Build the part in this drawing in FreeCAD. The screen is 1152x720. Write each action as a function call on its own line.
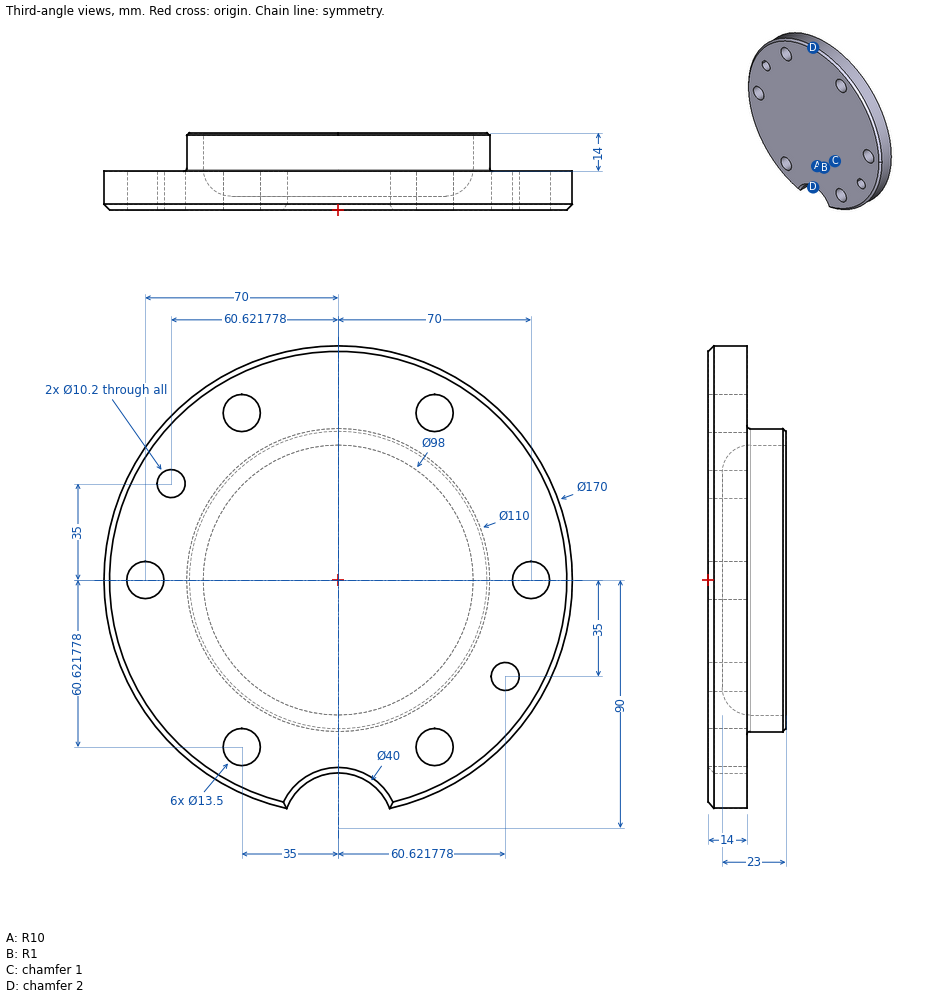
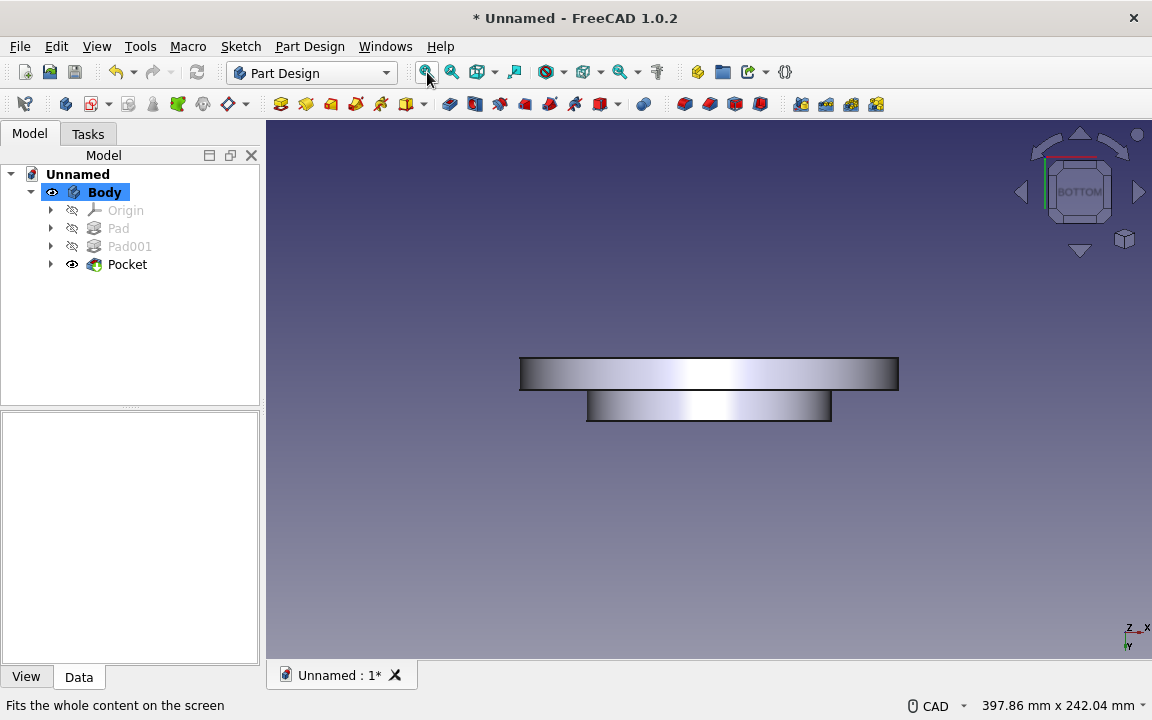
click(427, 72)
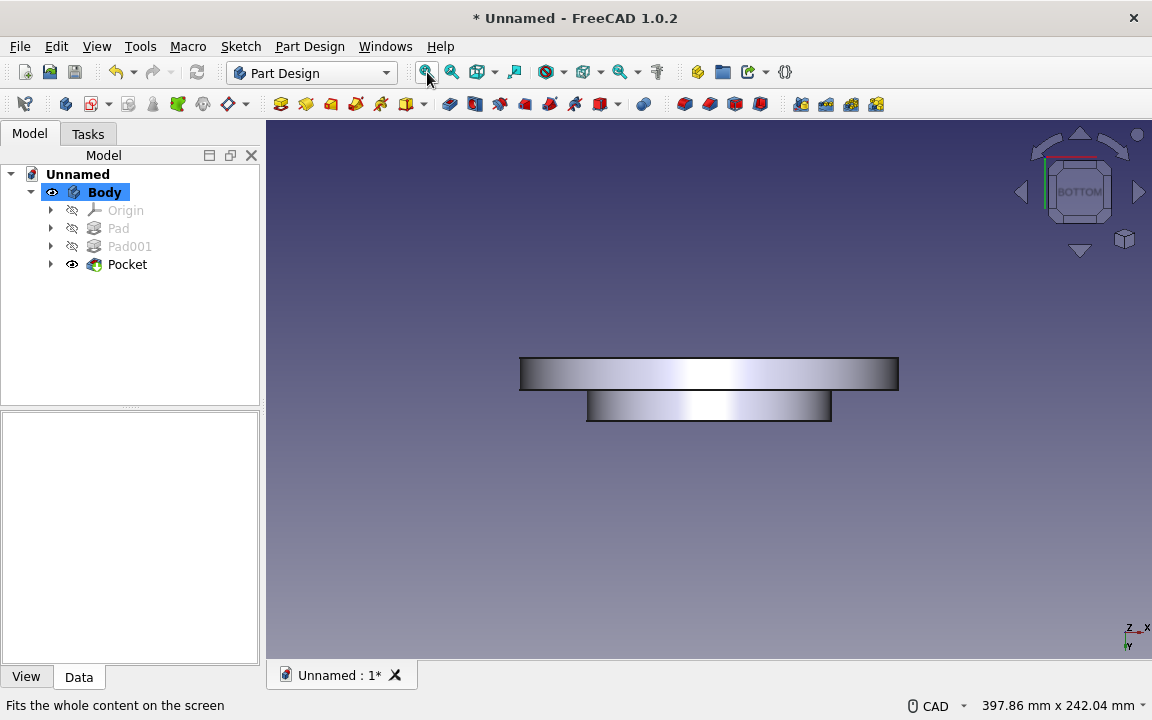
key(4)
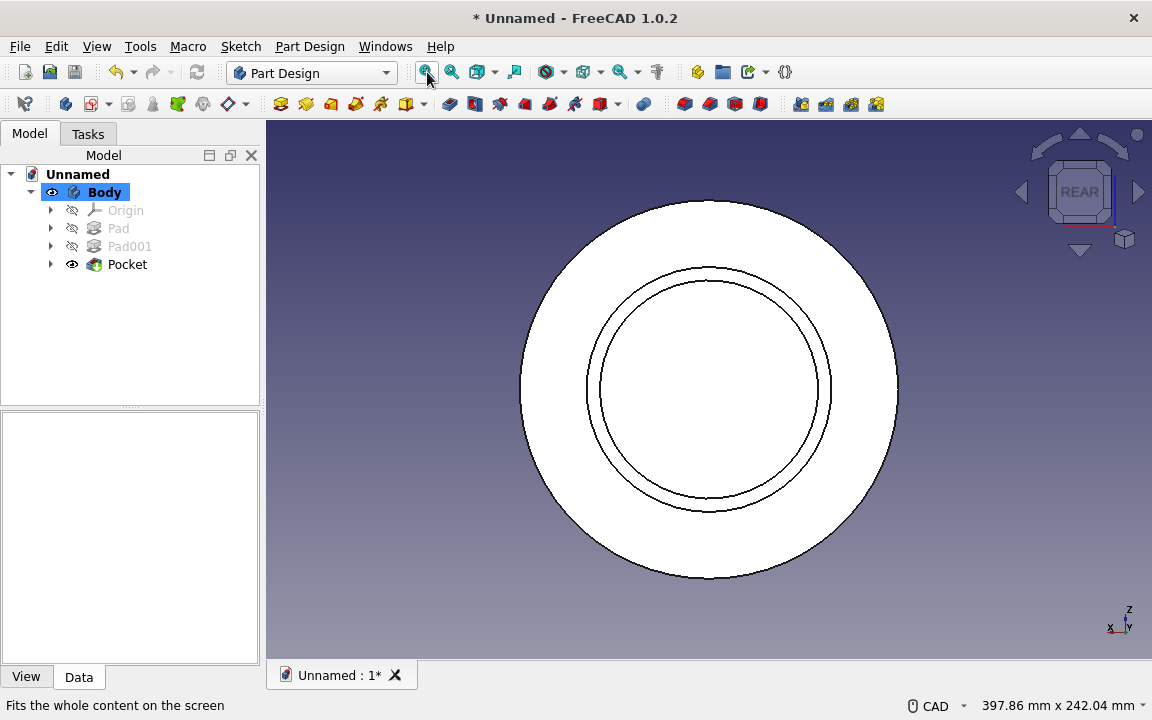
key(6)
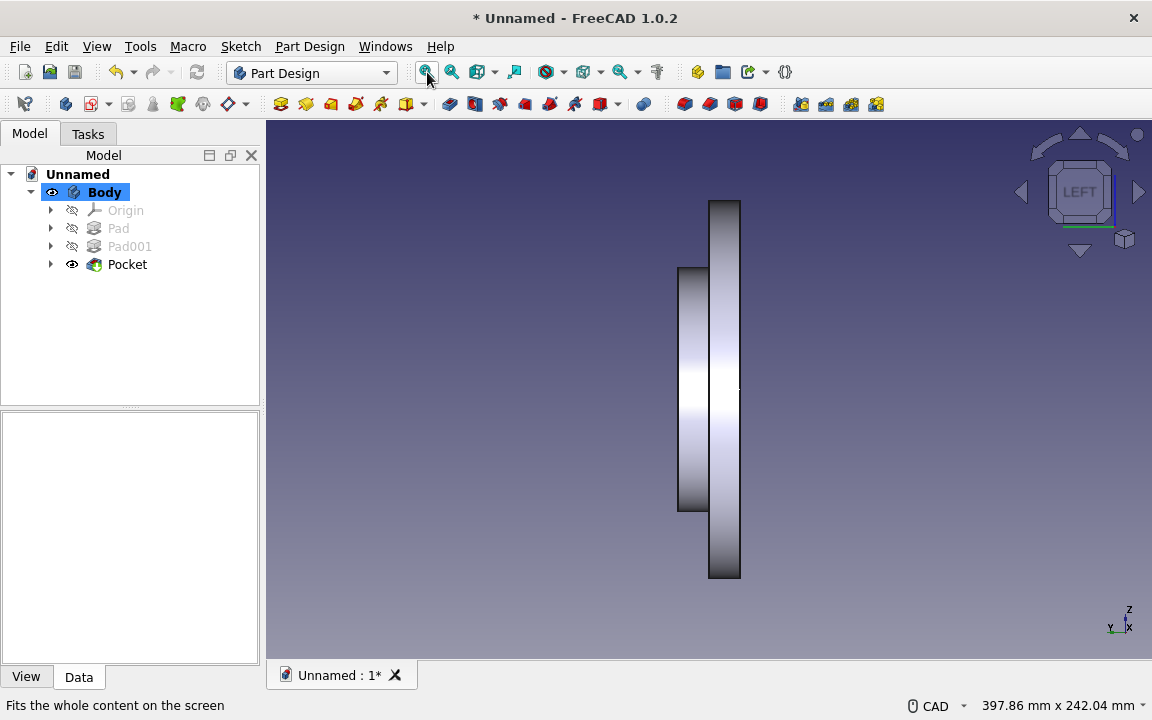
key(v)
key(3)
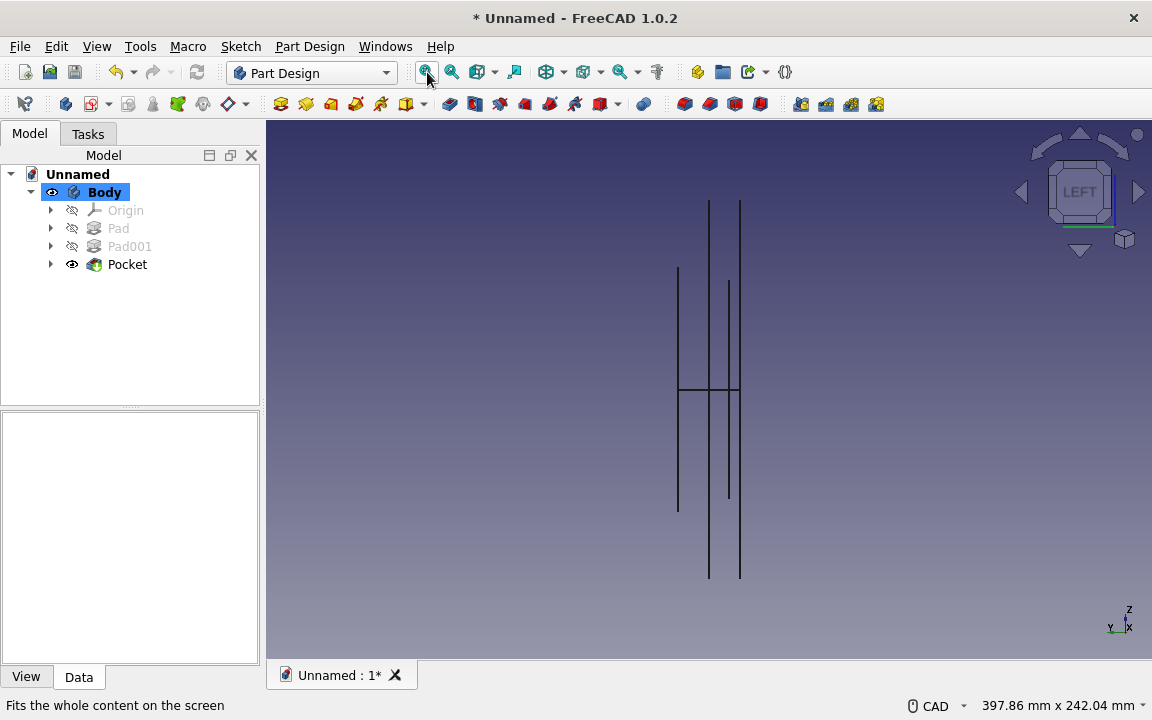
key(0)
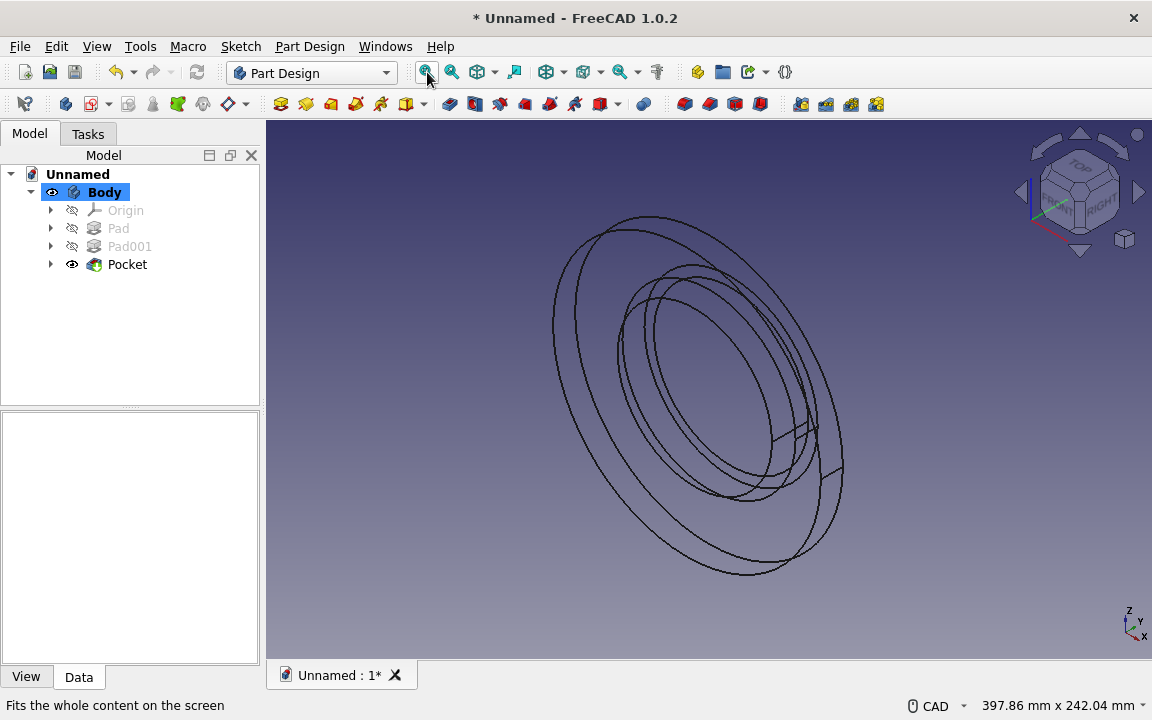
click(618, 352)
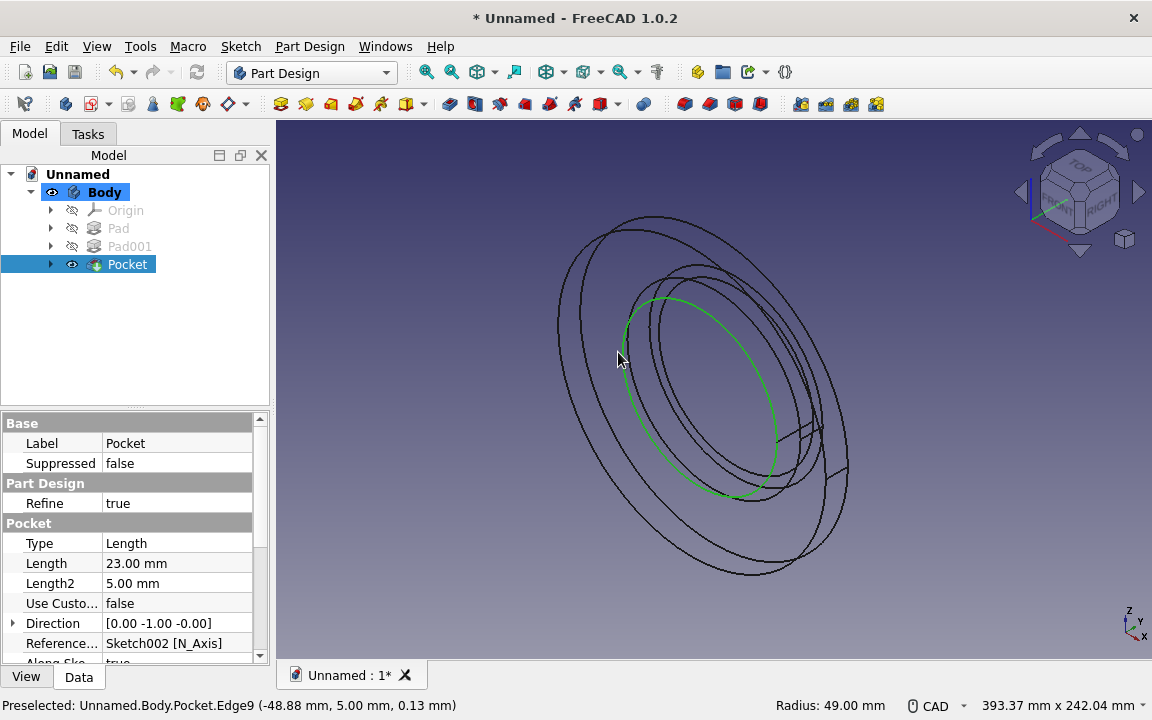
key(v)
key(1)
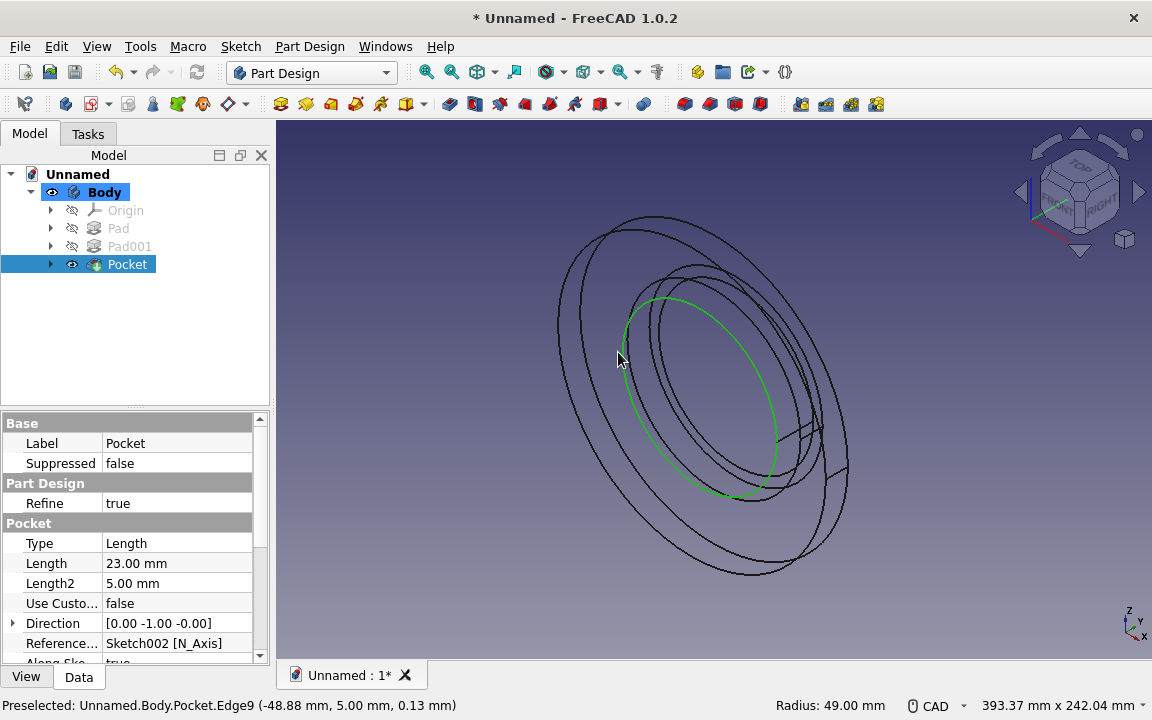
click(685, 104)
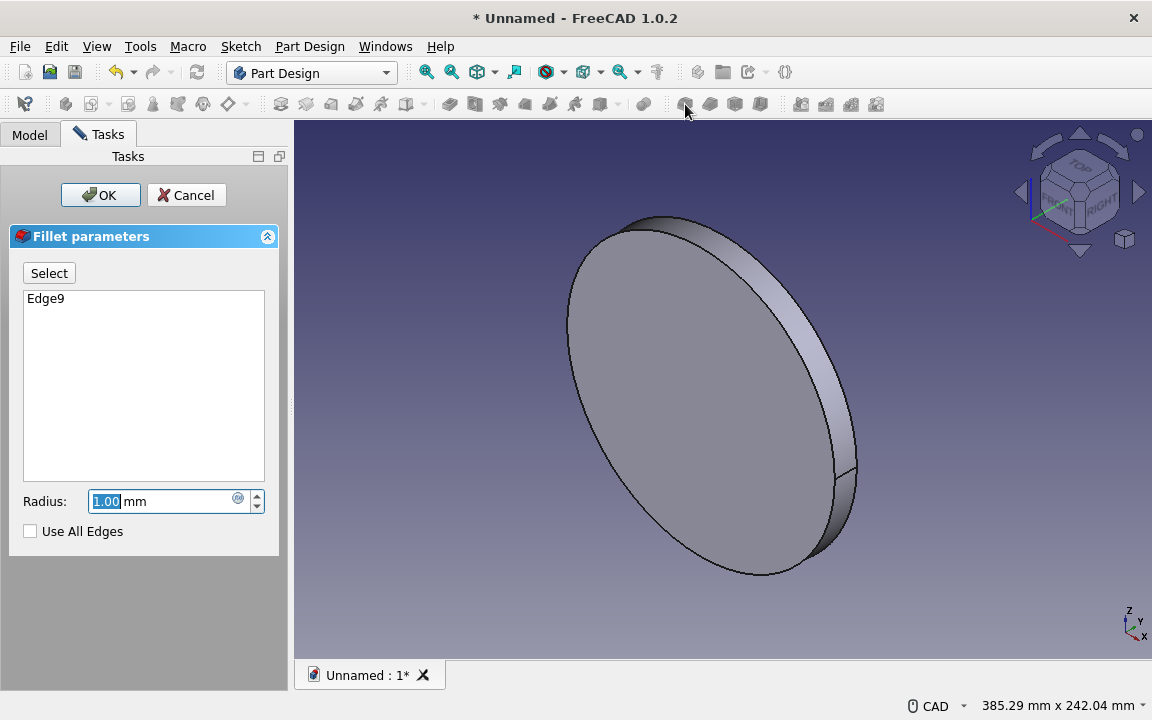
text(10)
key(Tab)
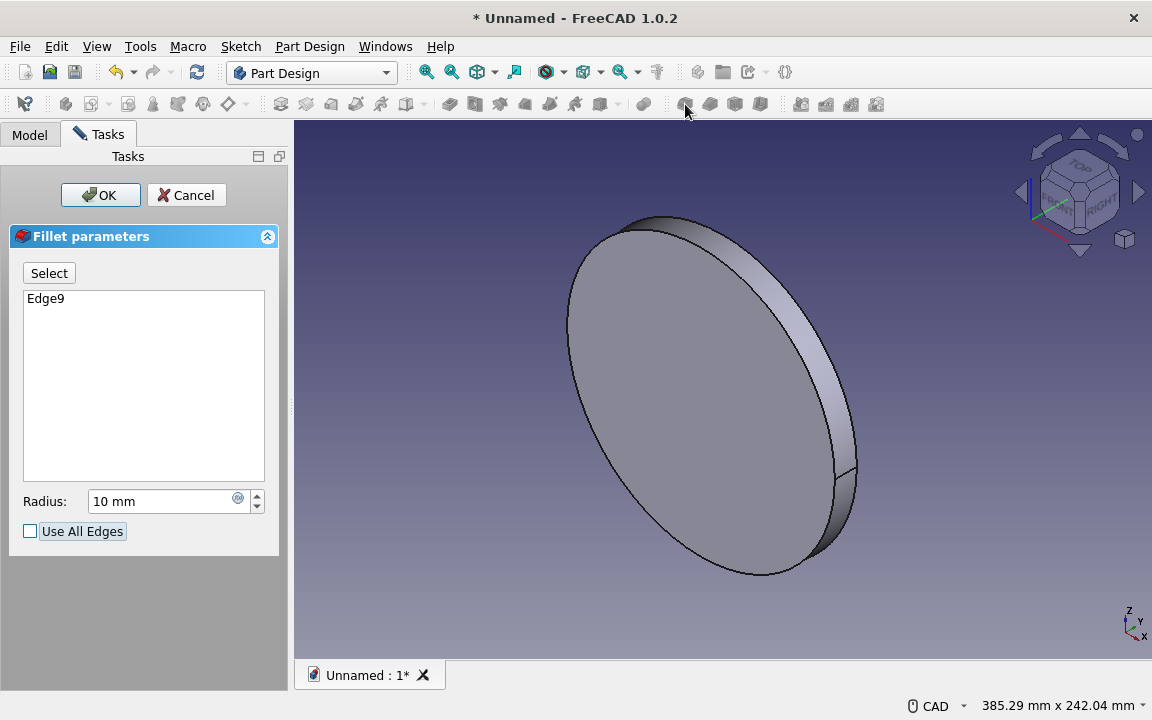
click(101, 195)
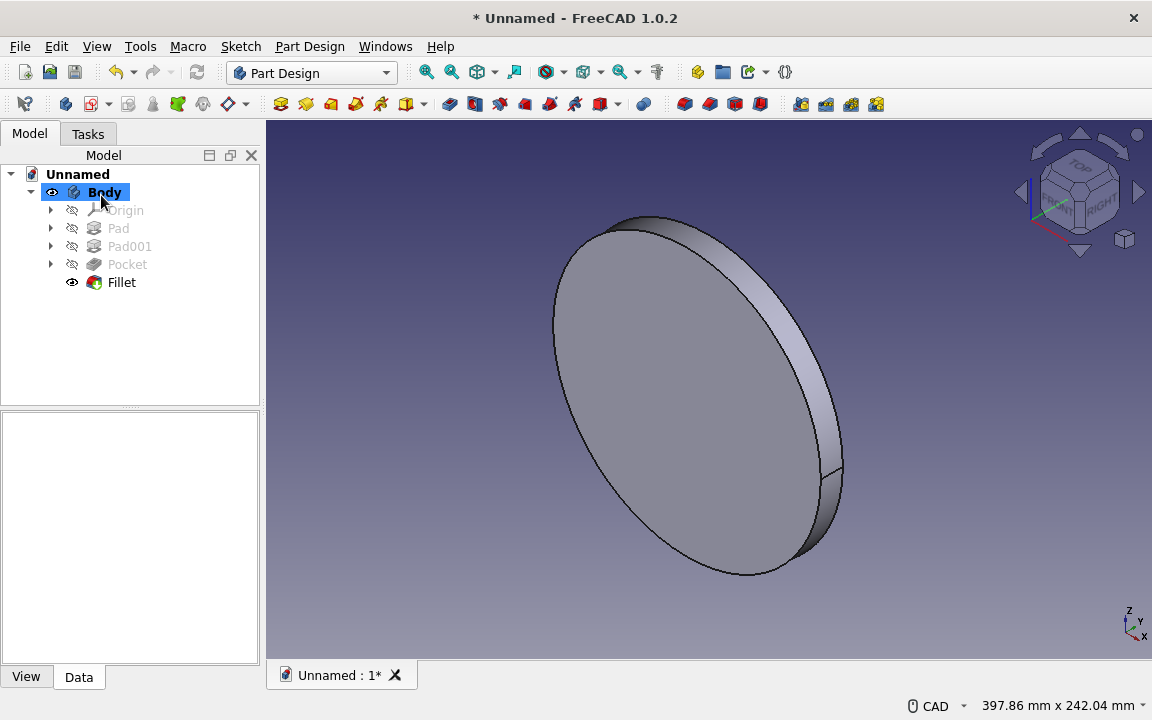
key(2)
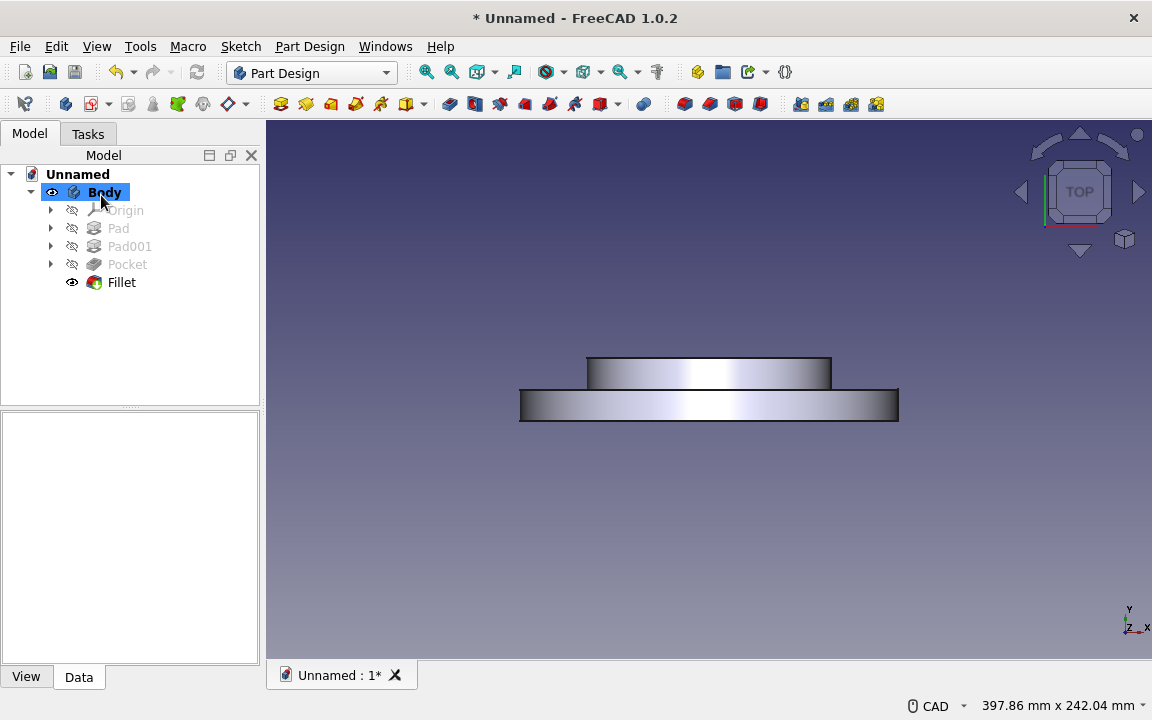
click(427, 72)